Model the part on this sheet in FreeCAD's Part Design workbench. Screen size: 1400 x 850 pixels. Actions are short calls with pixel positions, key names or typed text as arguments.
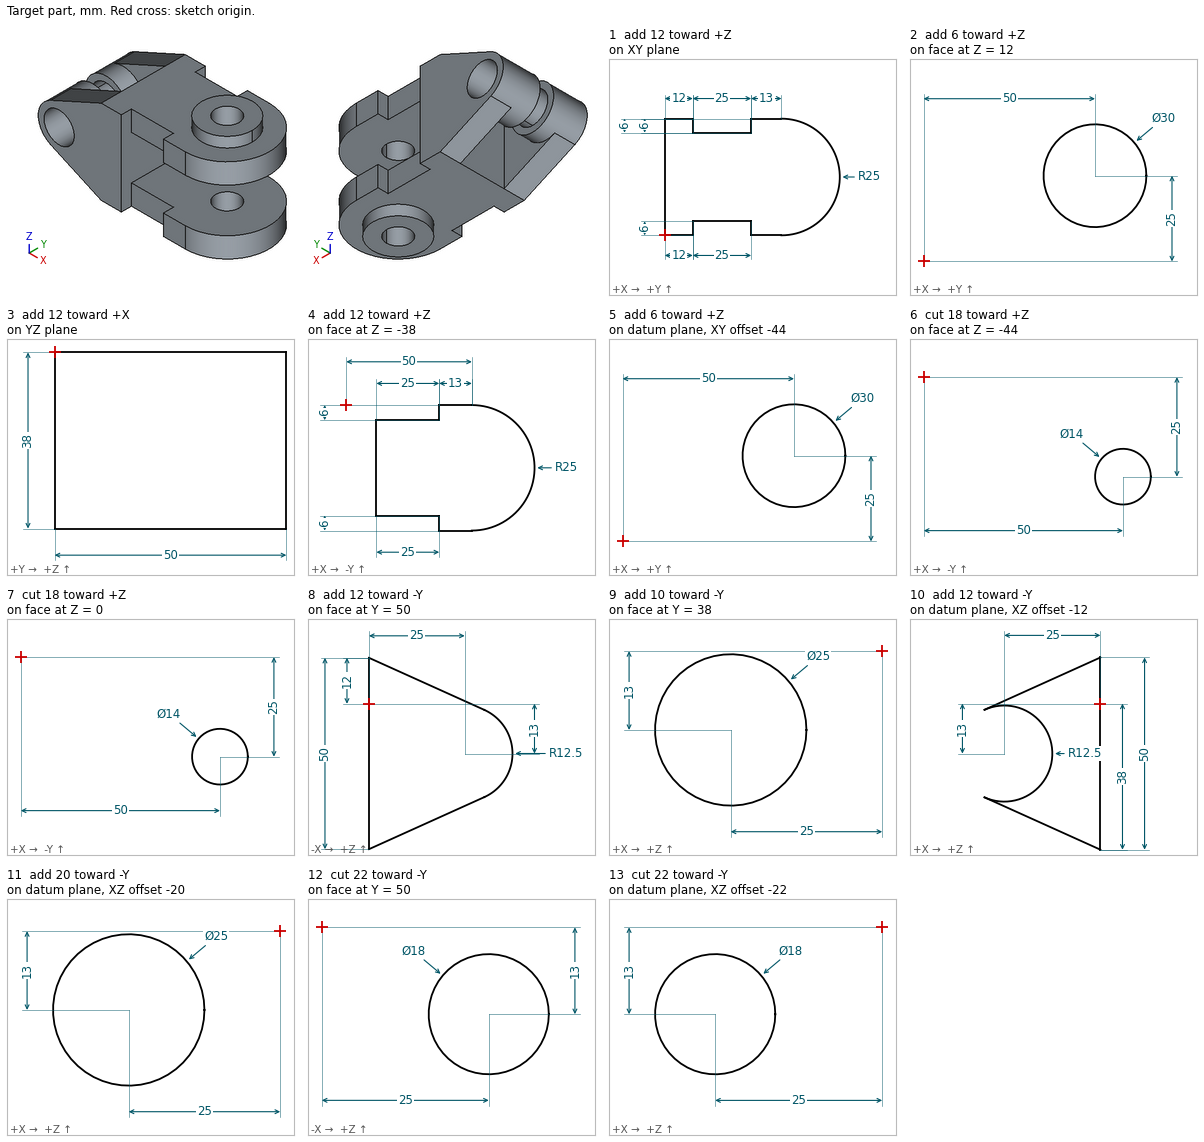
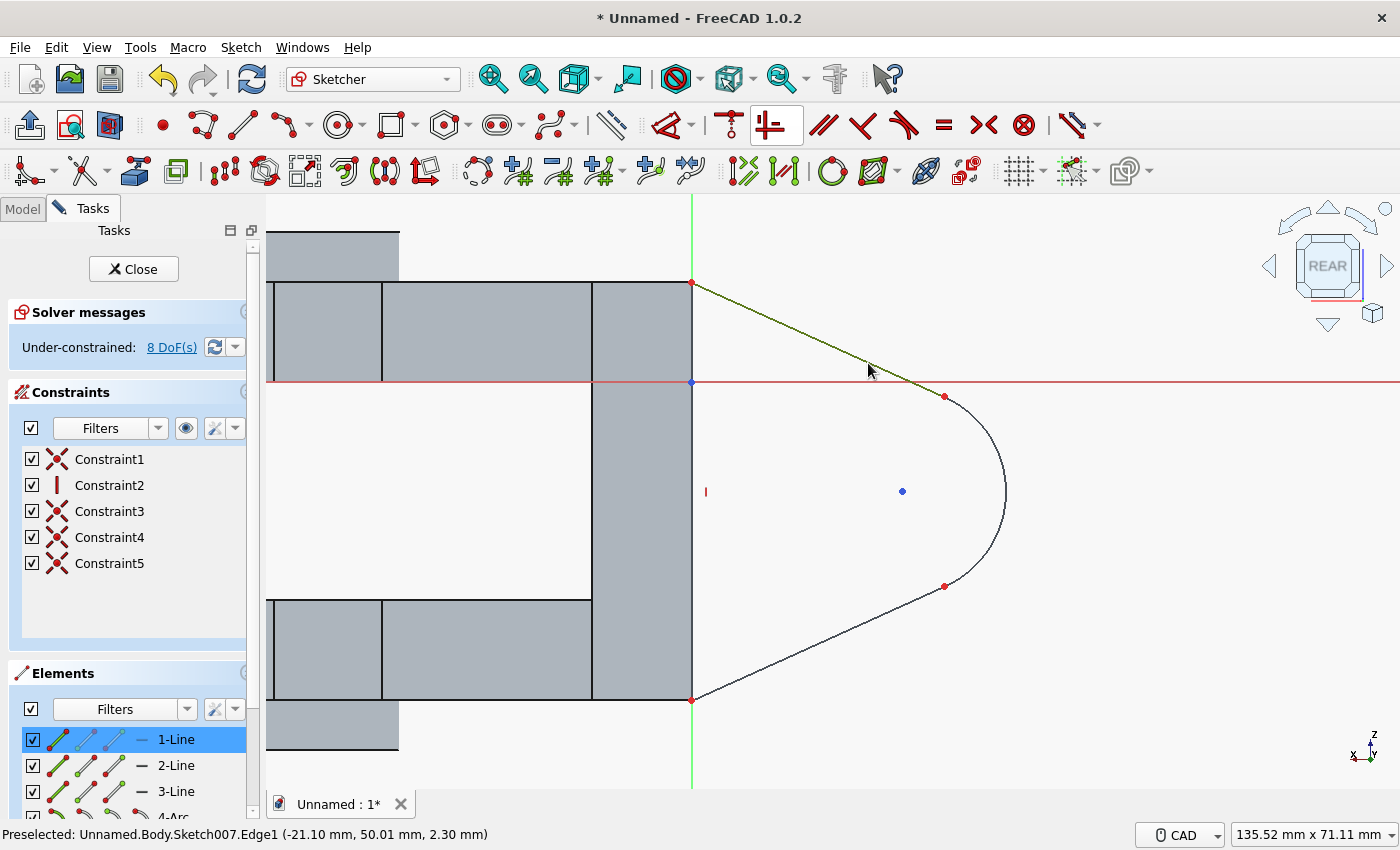
click(995, 538)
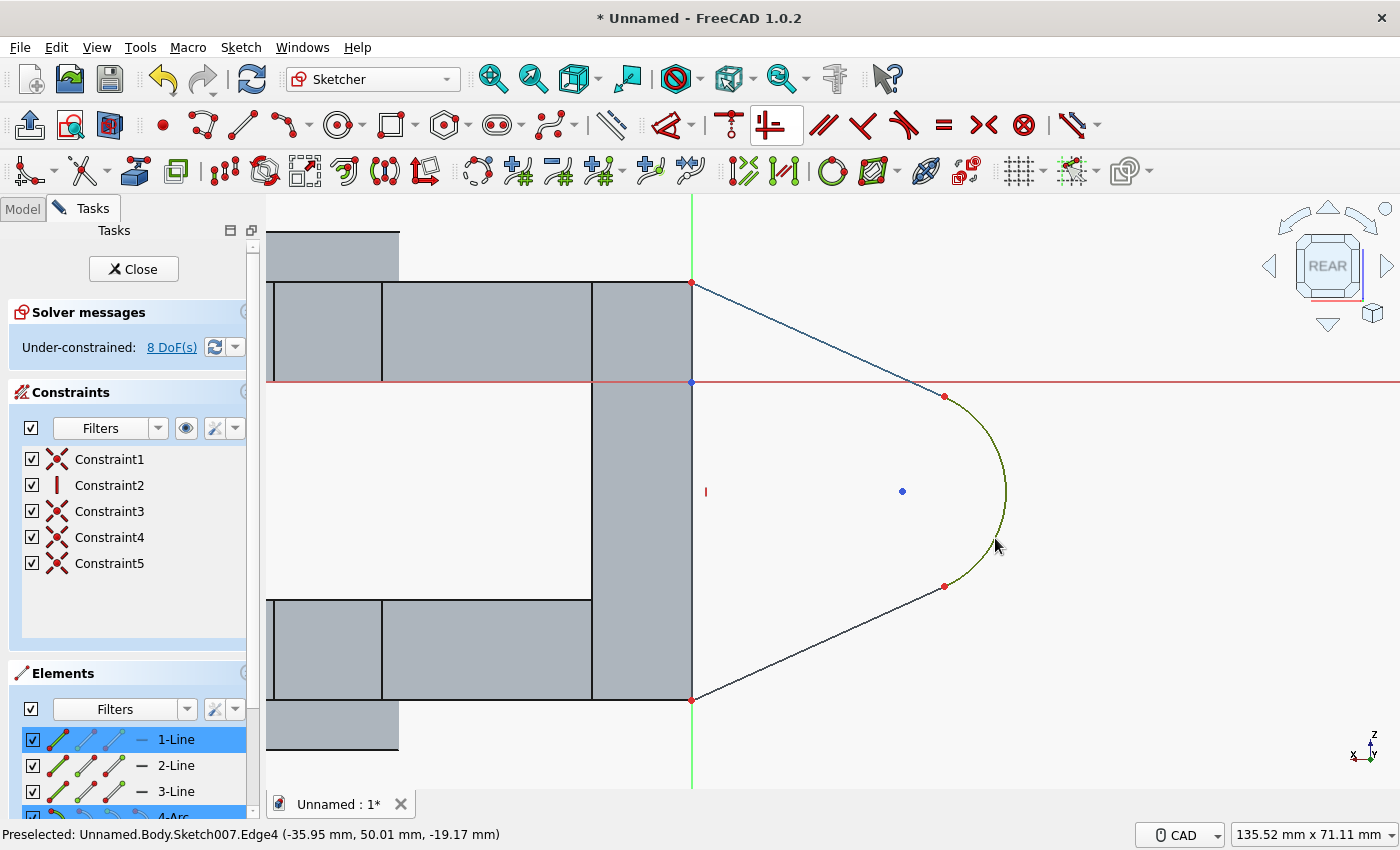
click(904, 126)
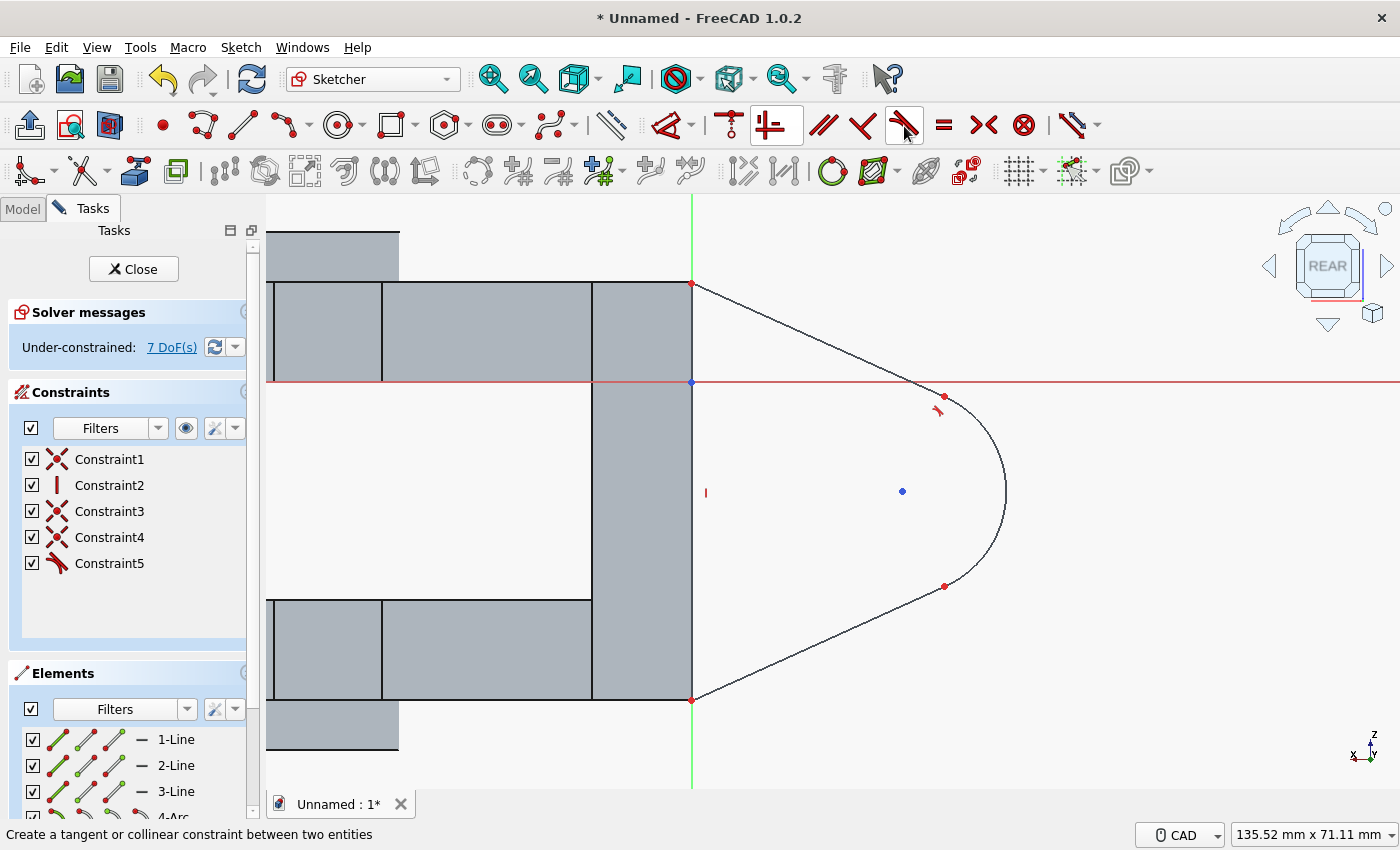
click(768, 667)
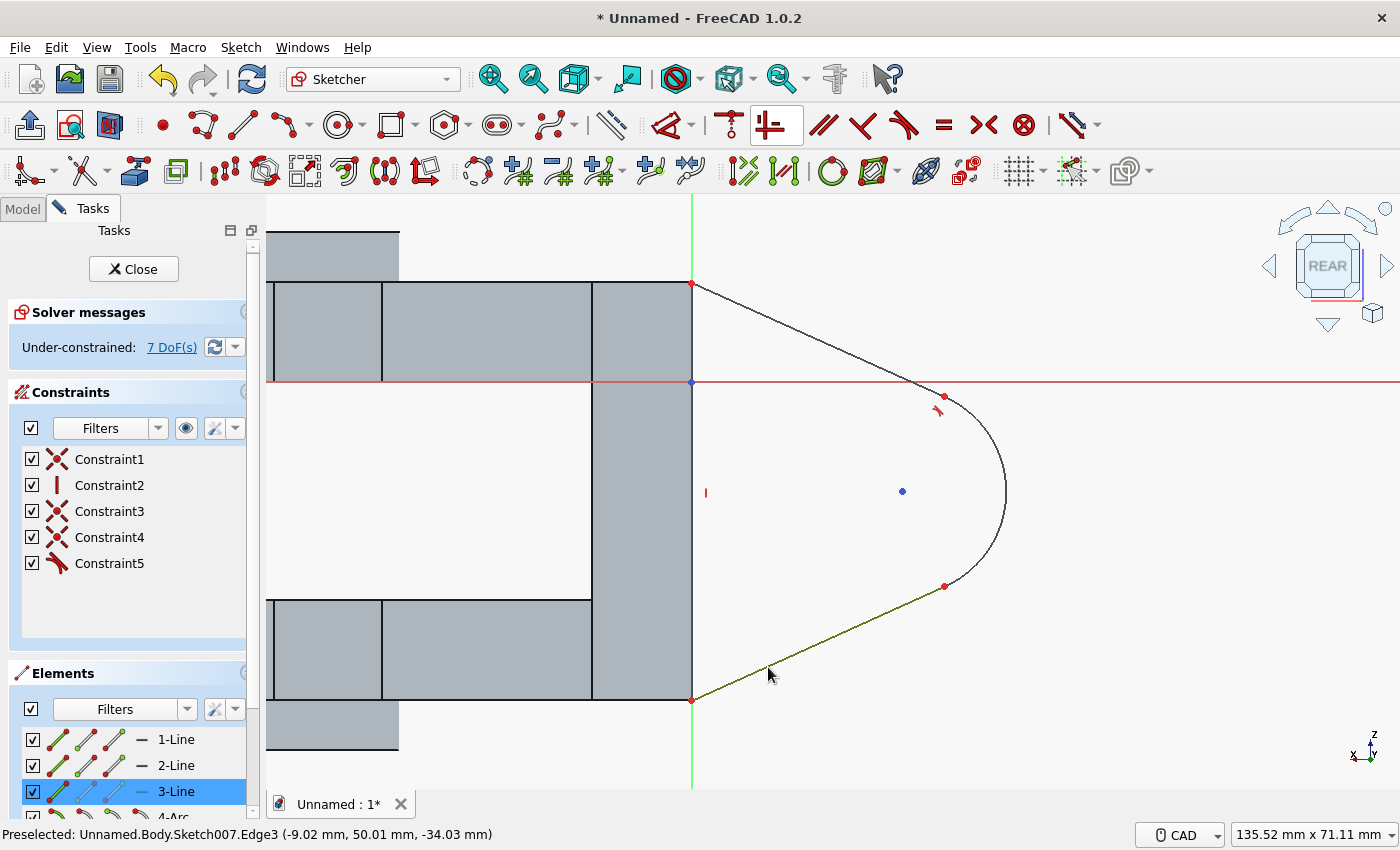
click(995, 538)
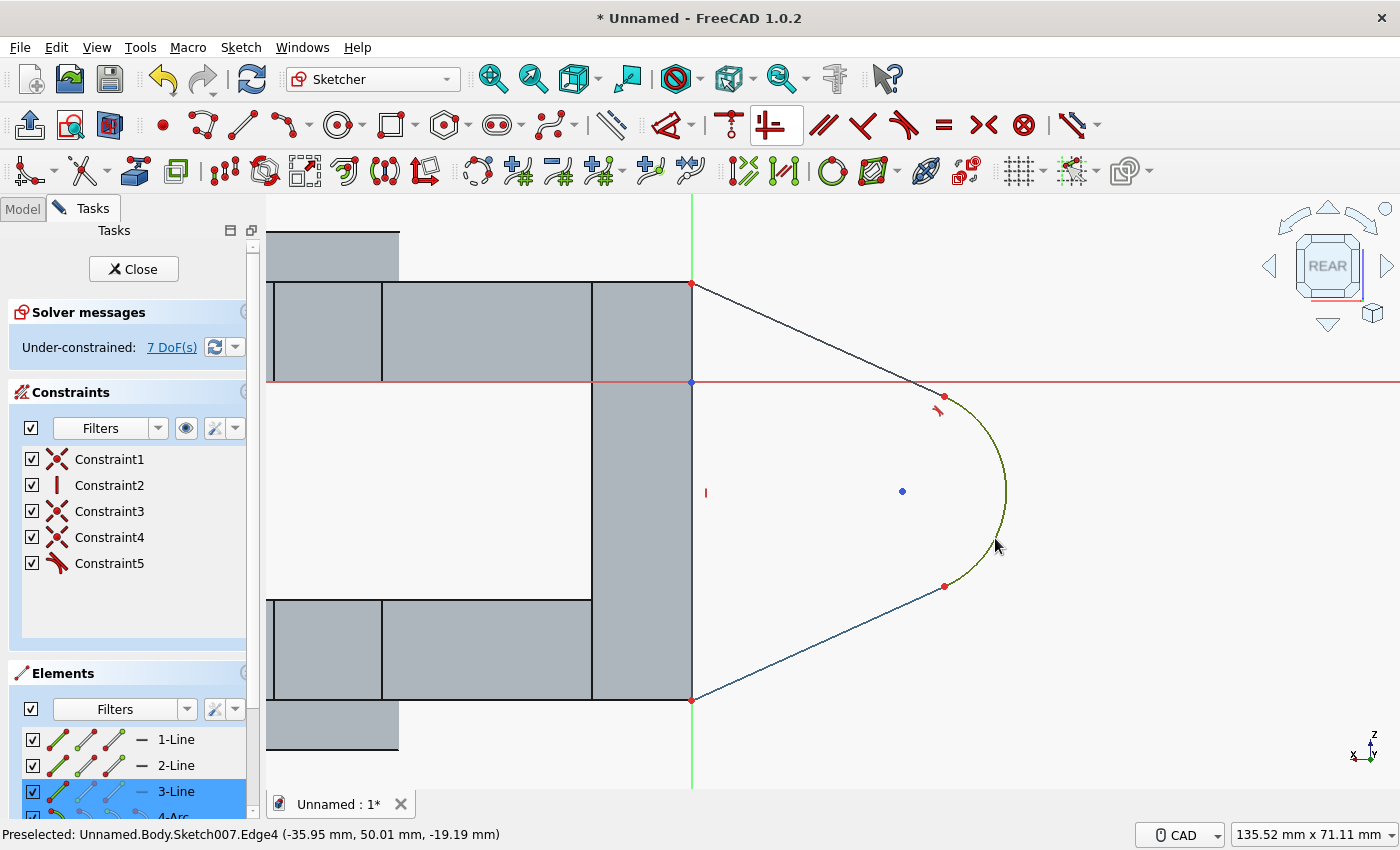
key(t)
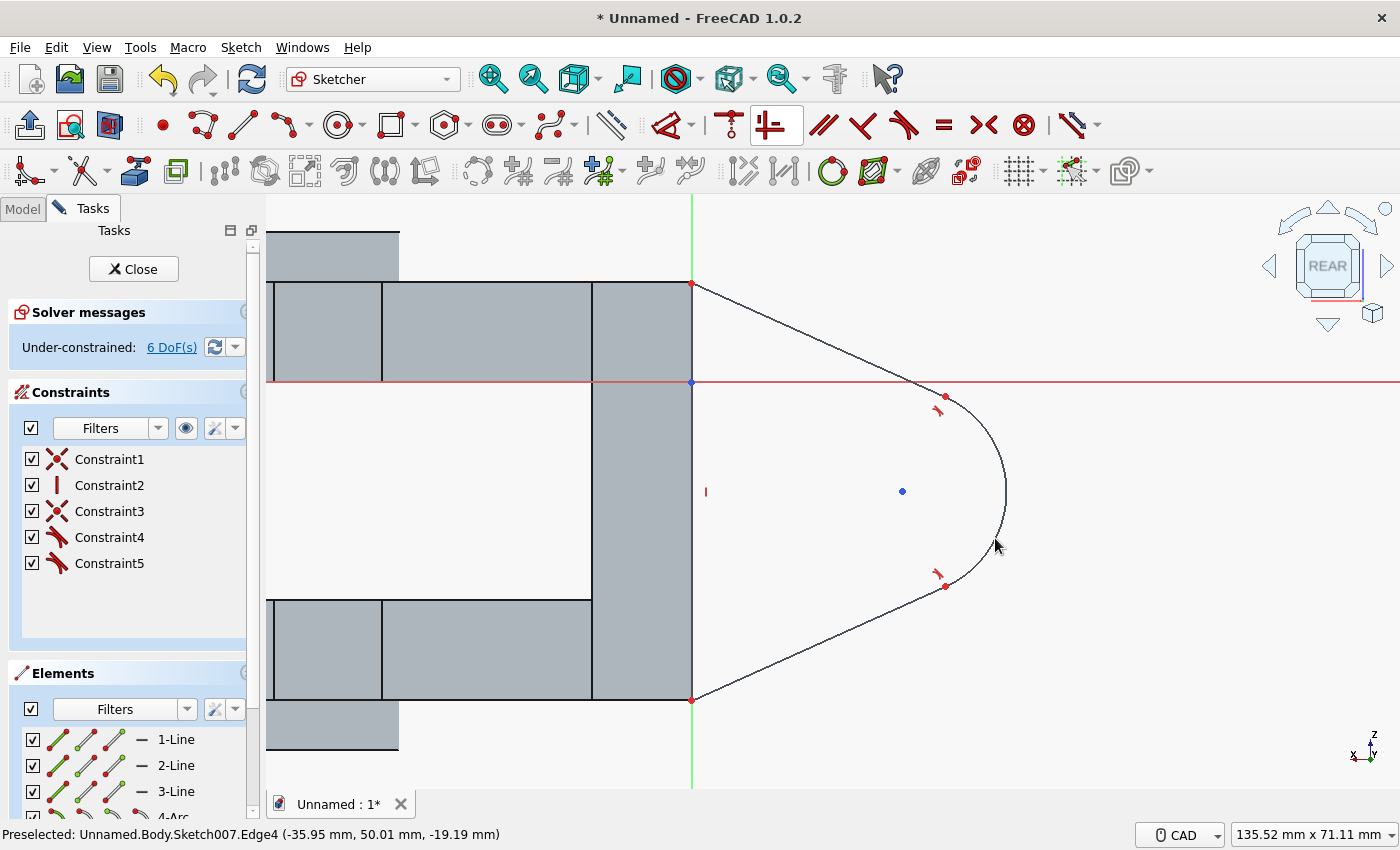
key(d)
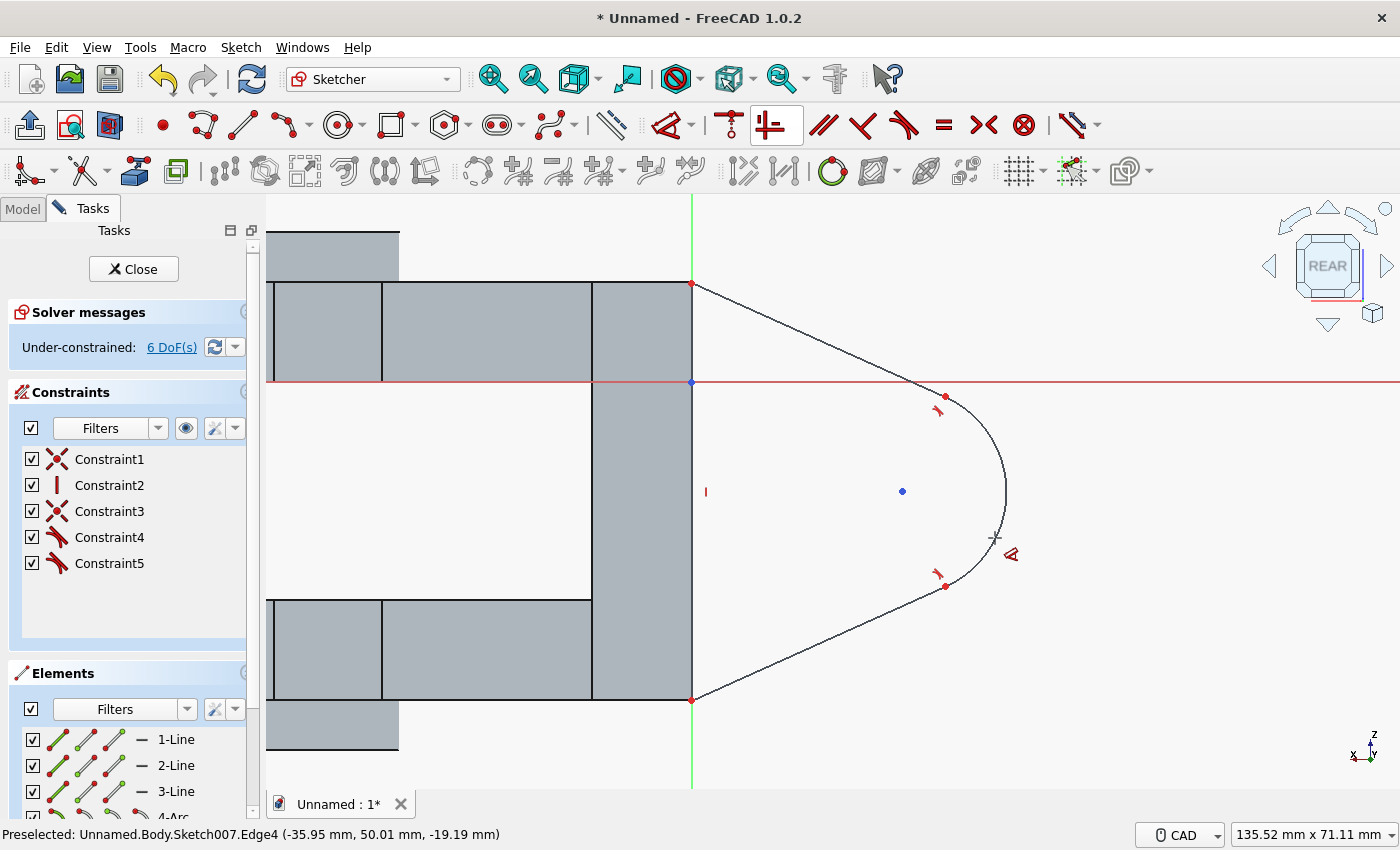
click(996, 538)
click(1025, 552)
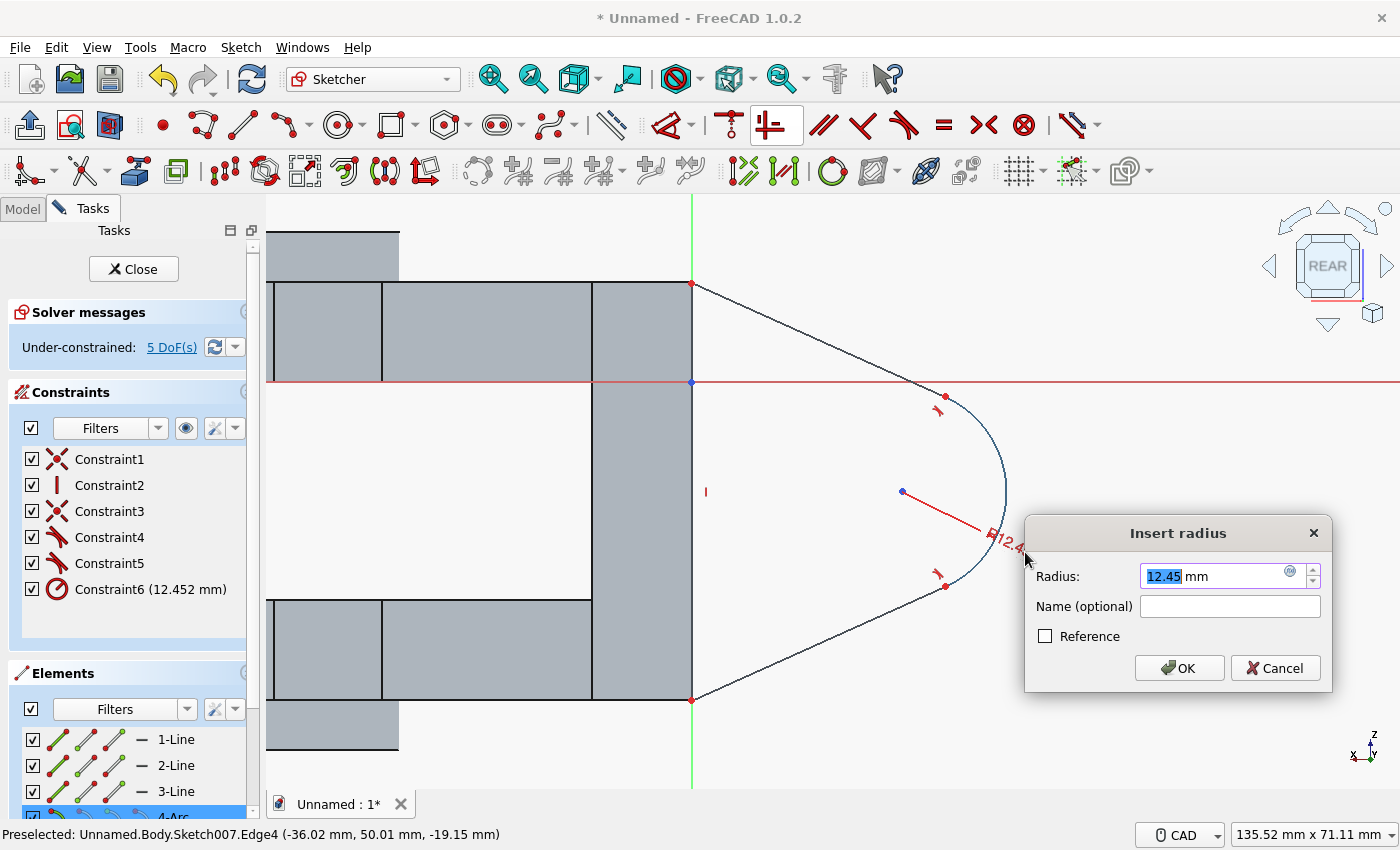
text(12.5)
key(Return)
key(Escape)